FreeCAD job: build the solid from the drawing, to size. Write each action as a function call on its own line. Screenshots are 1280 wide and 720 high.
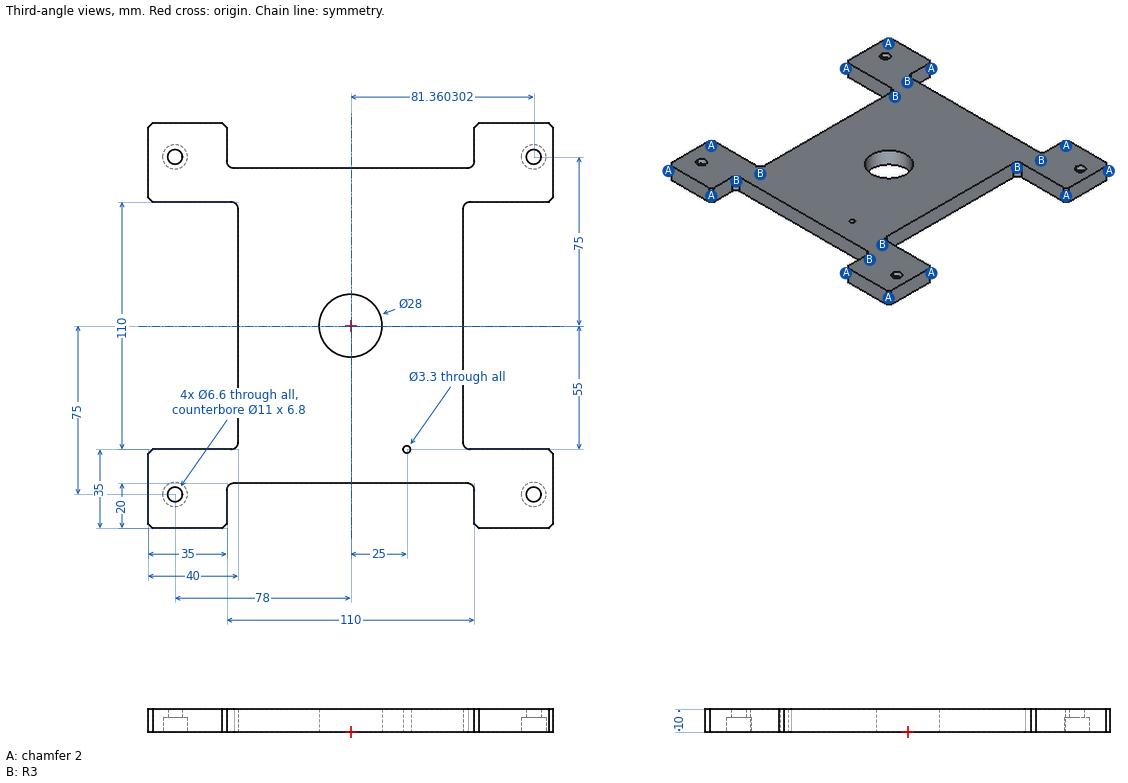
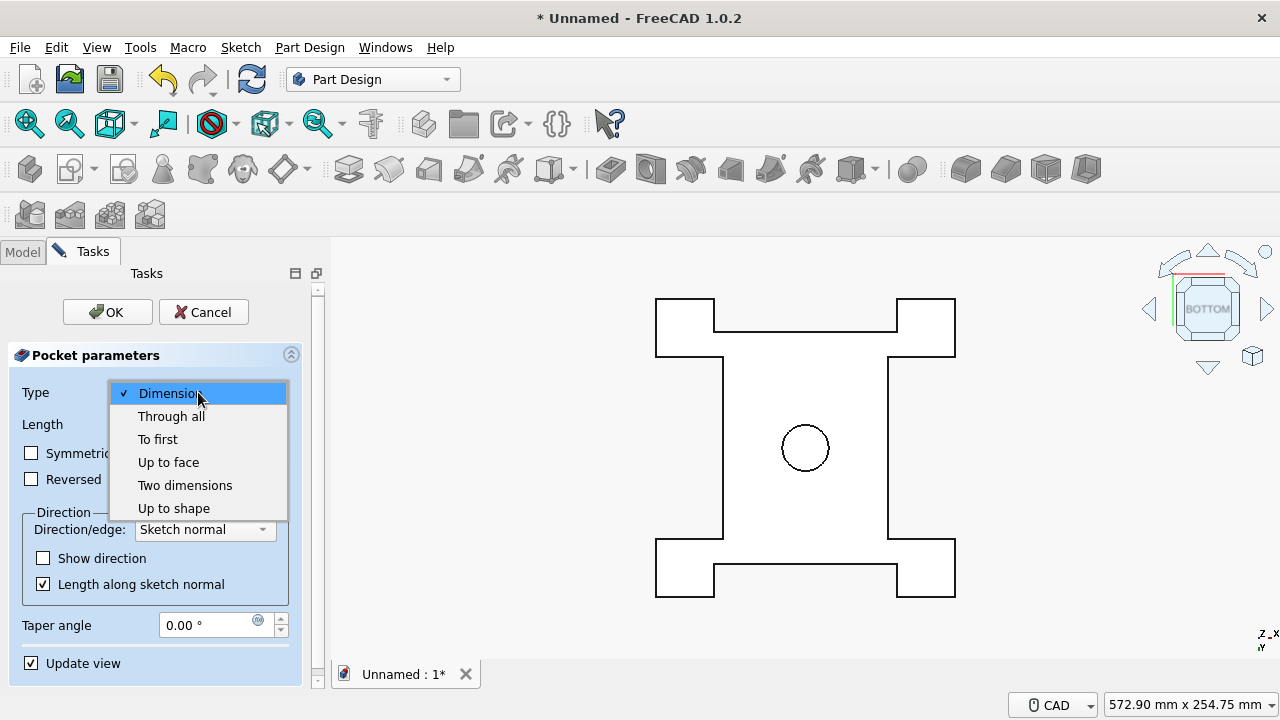
click(198, 416)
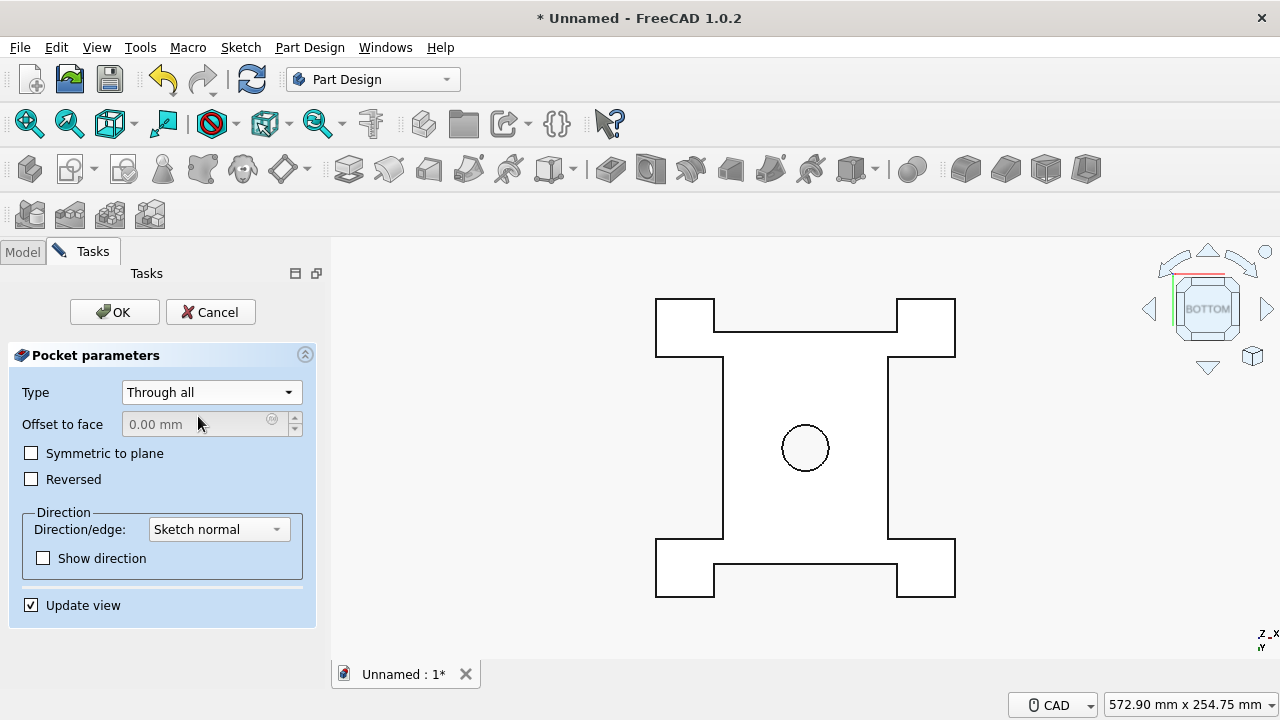
click(115, 312)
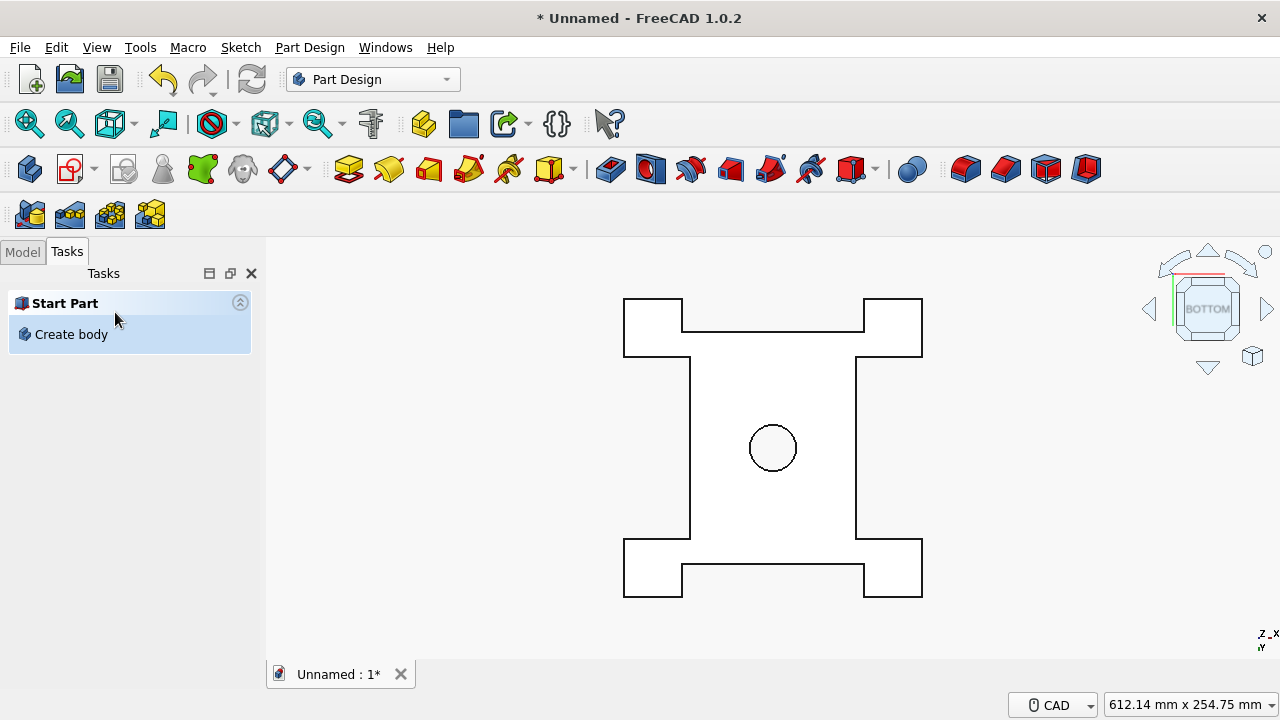
key(0)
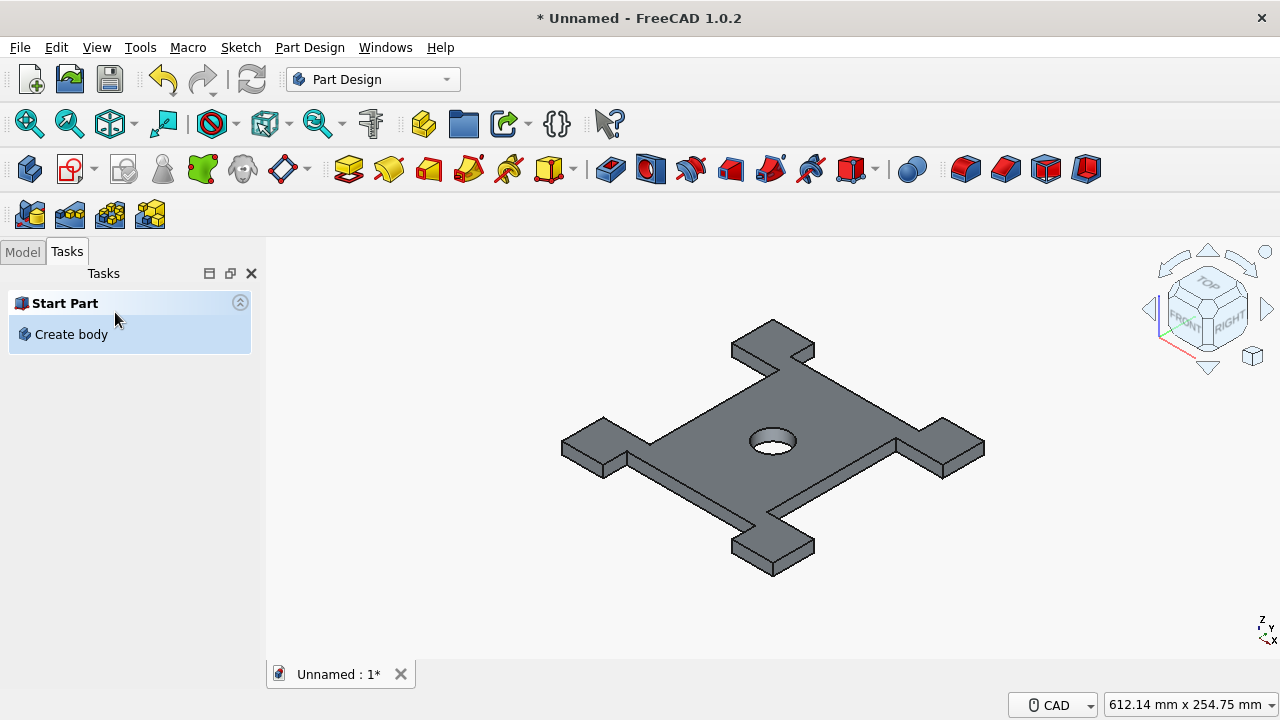
click(833, 440)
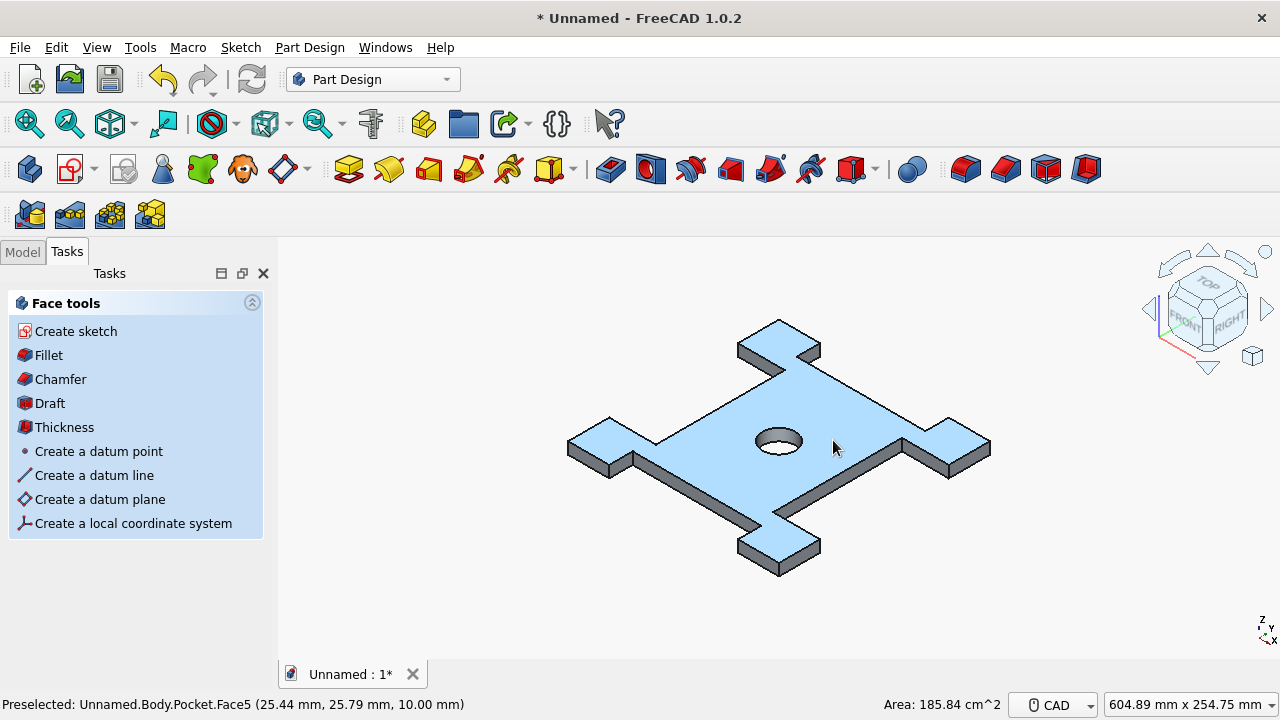
click(70, 170)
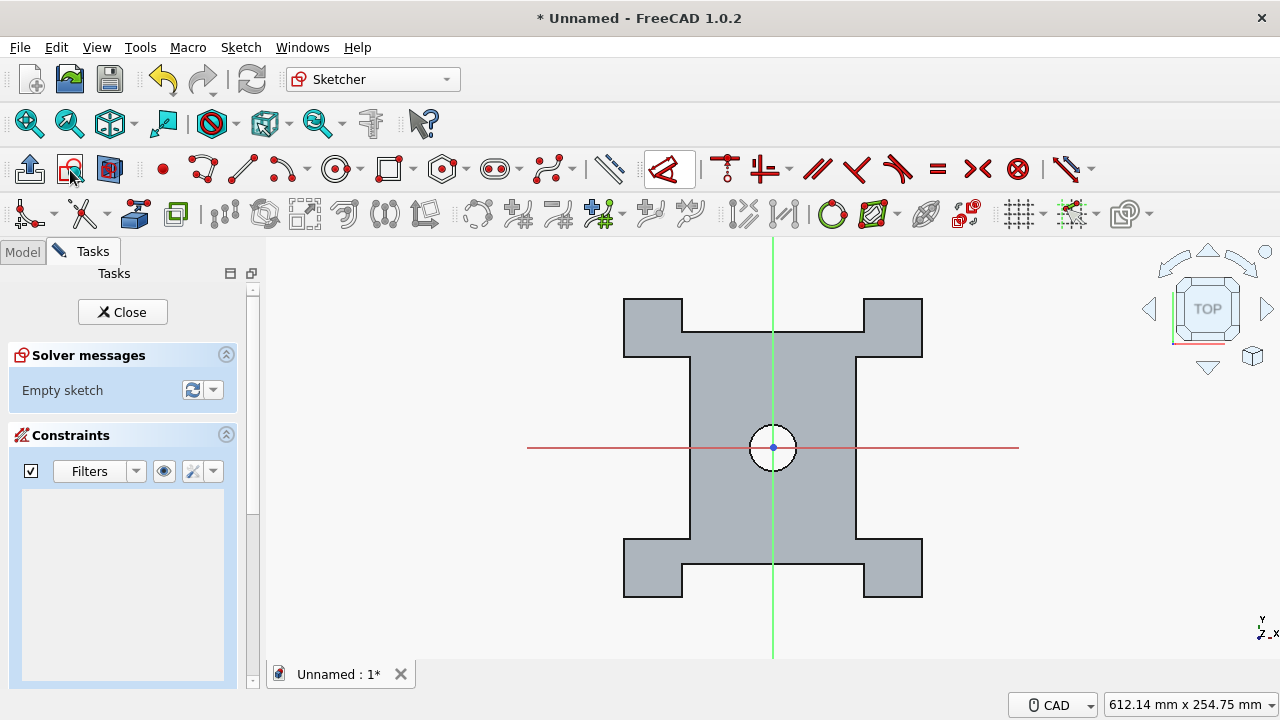
scroll(820, 544, up, 15)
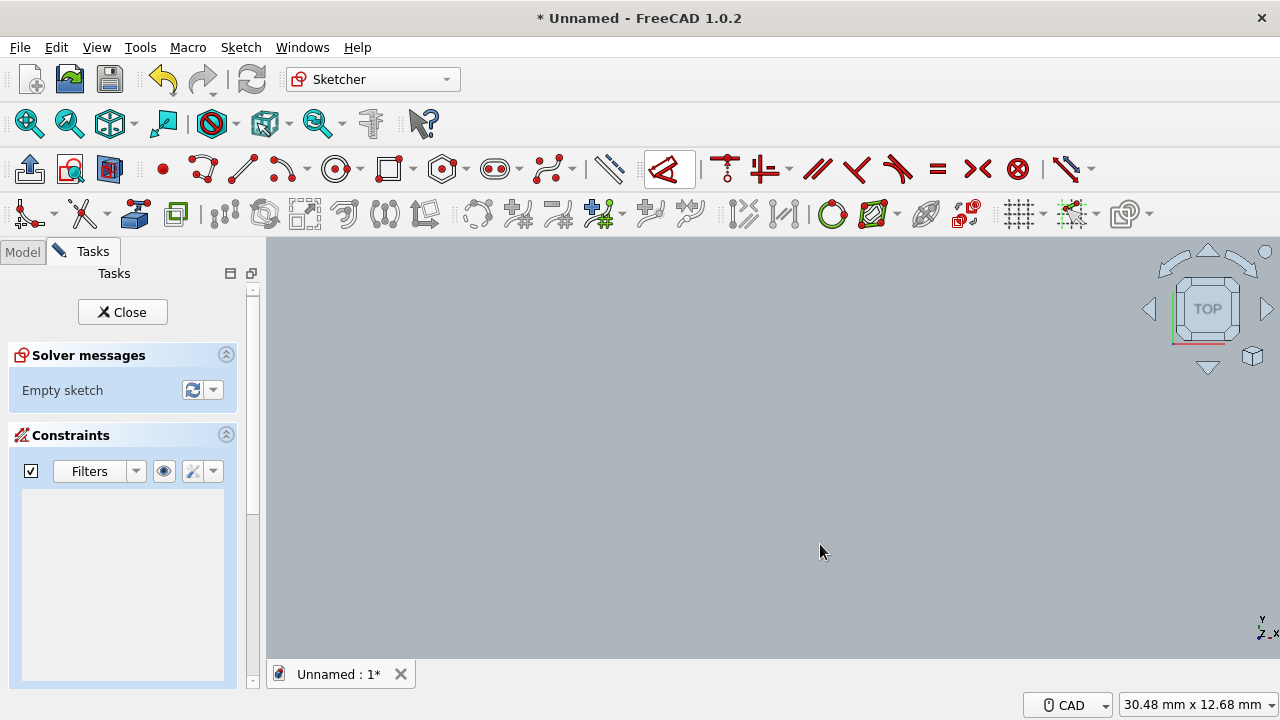
scroll(691, 419, up, 4)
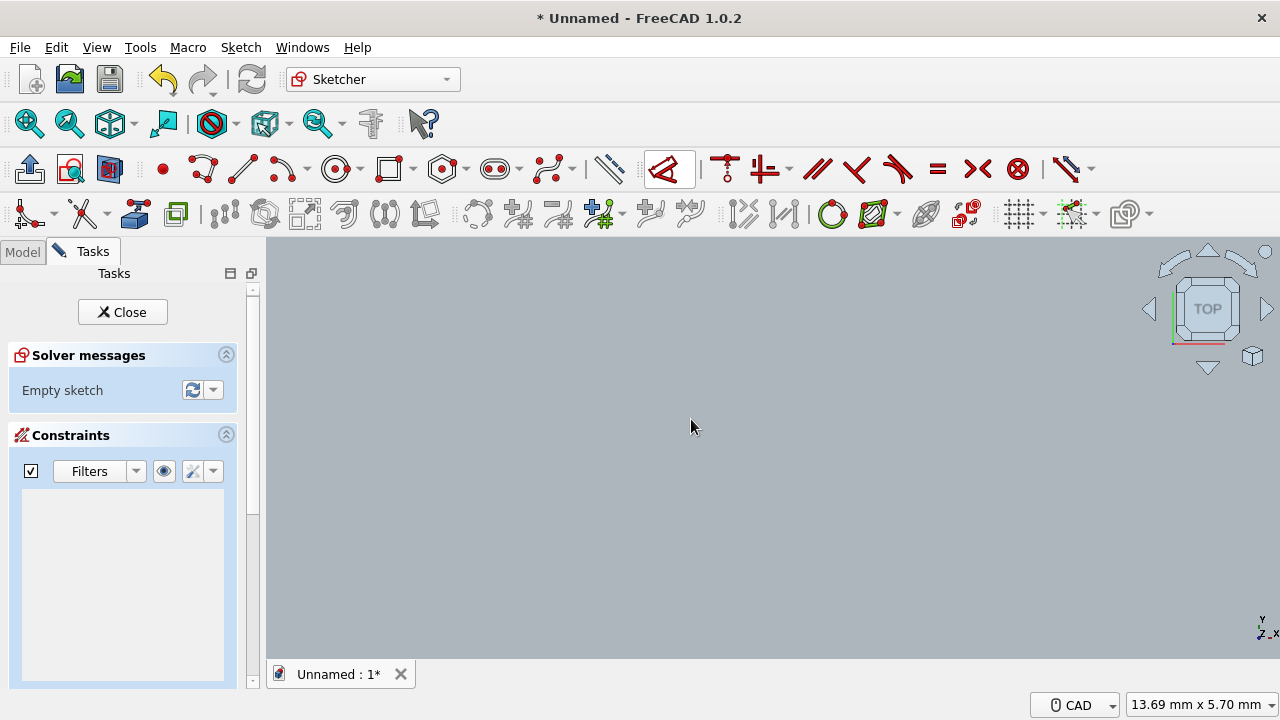
click(336, 170)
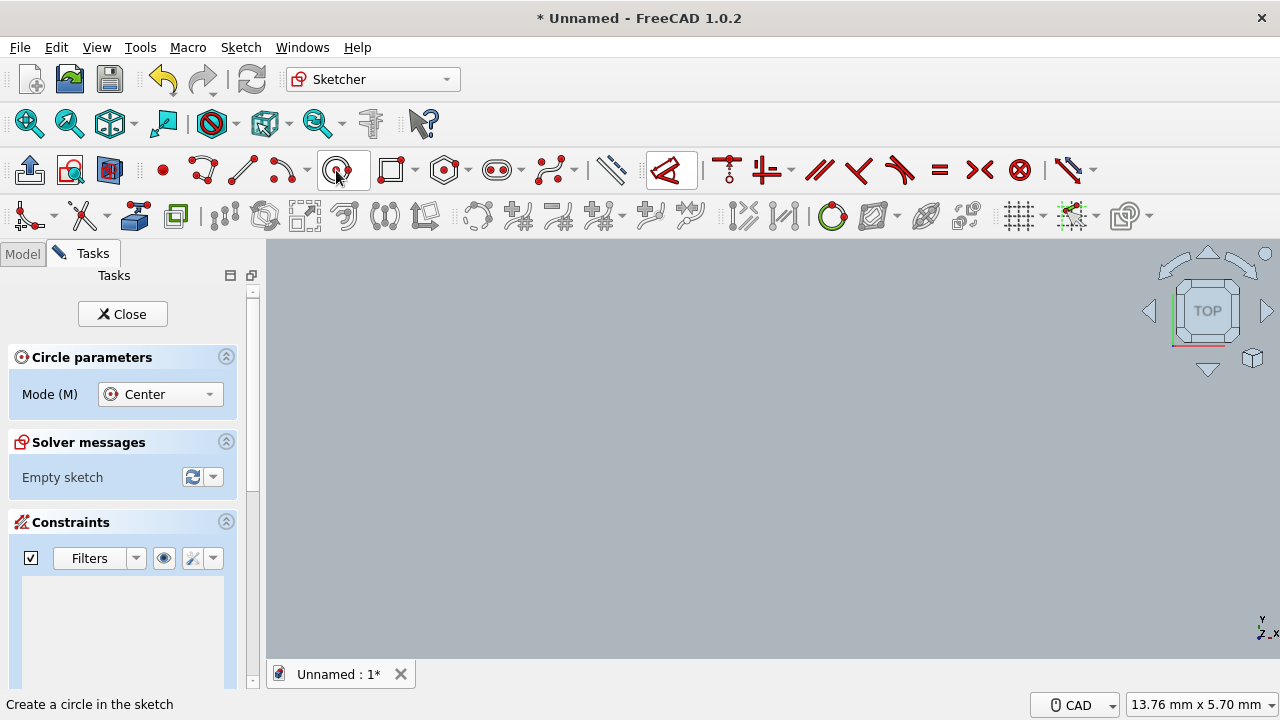
click(705, 448)
click(791, 362)
key(Escape)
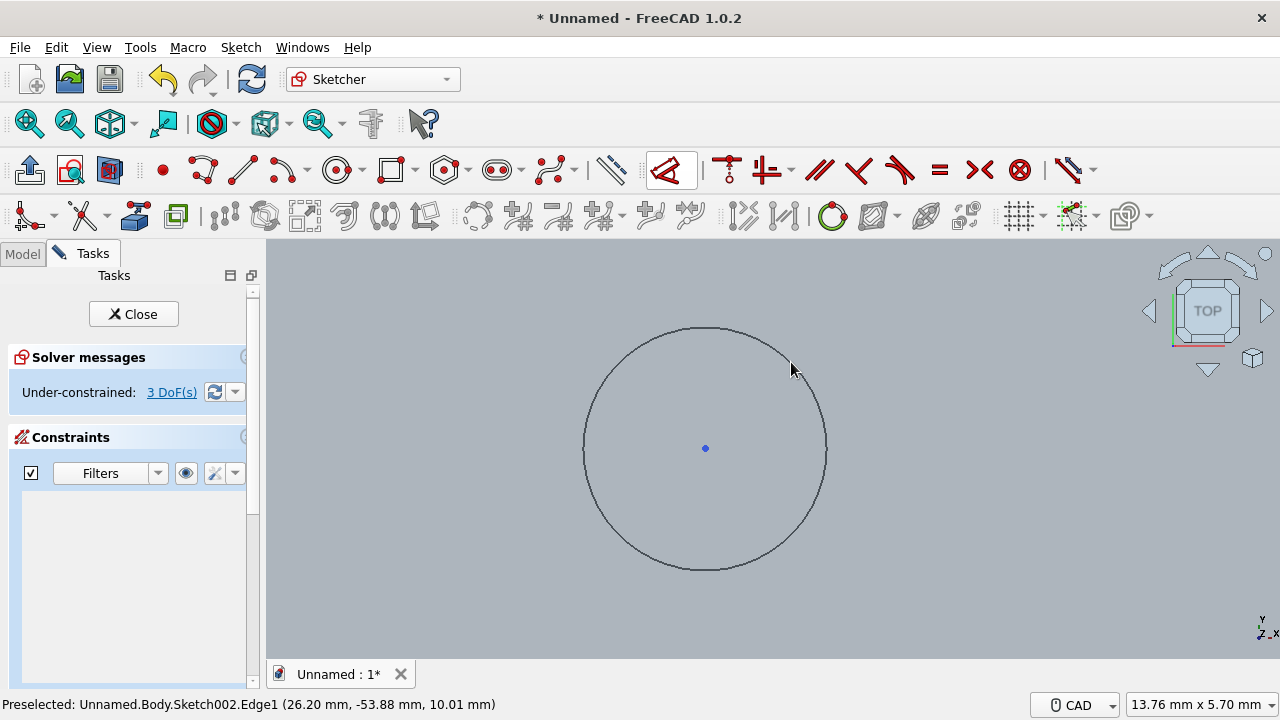
click(791, 363)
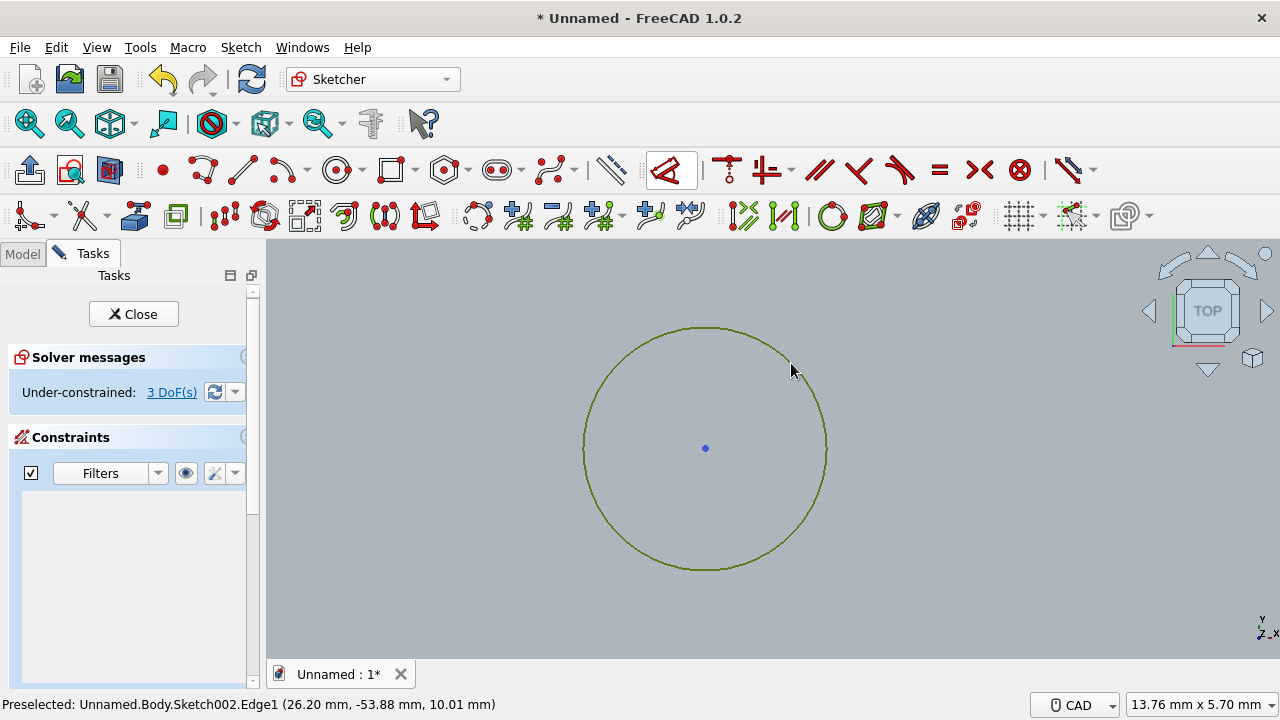
click(692, 170)